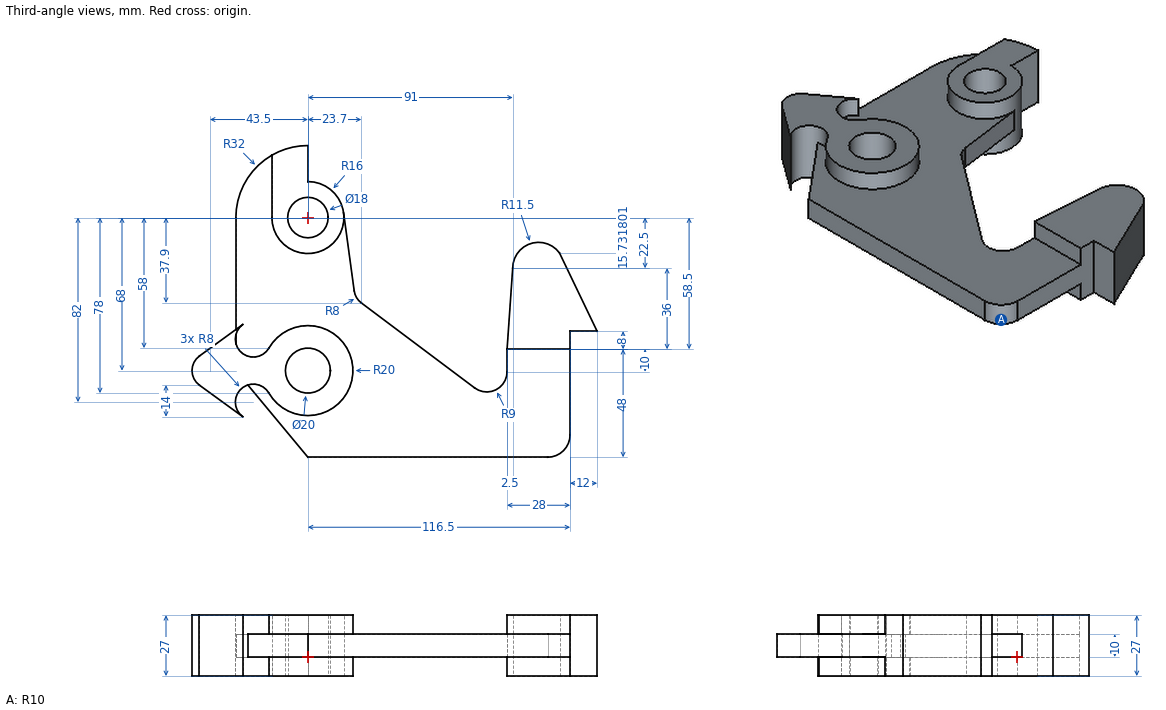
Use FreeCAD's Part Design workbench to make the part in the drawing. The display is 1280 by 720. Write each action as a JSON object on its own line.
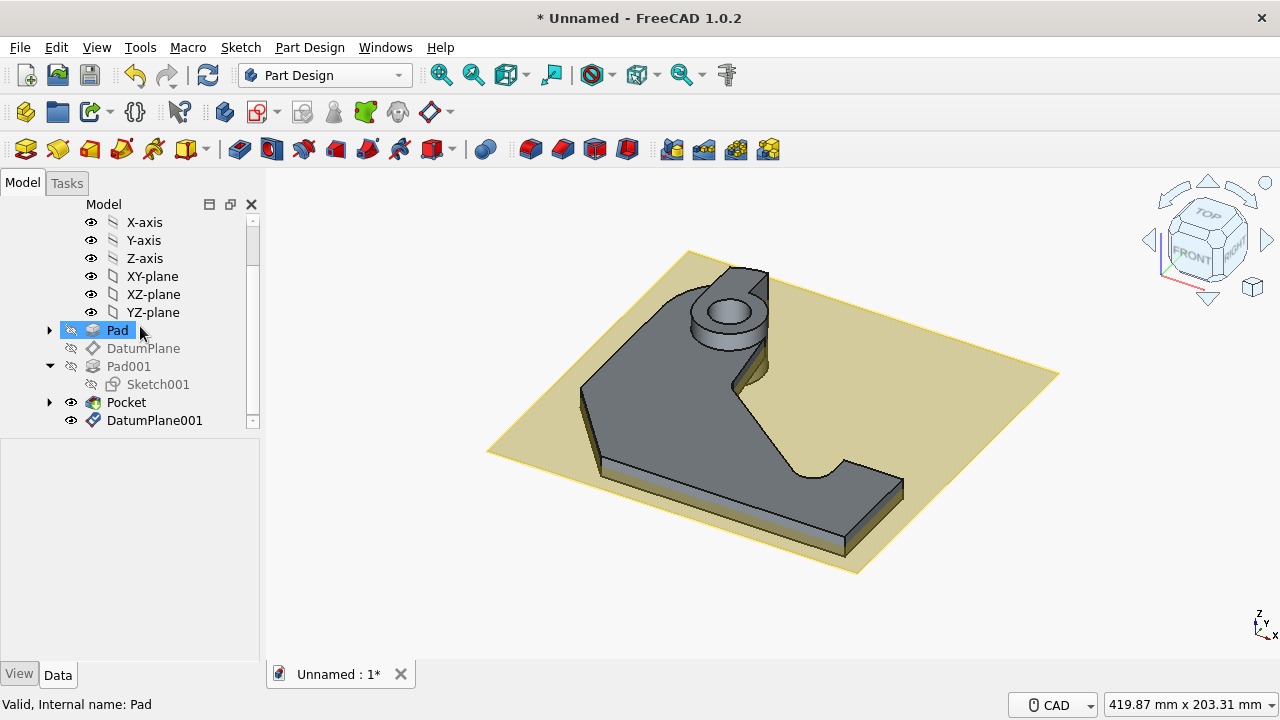
{"action": "left_click", "coordinate": [116, 420]}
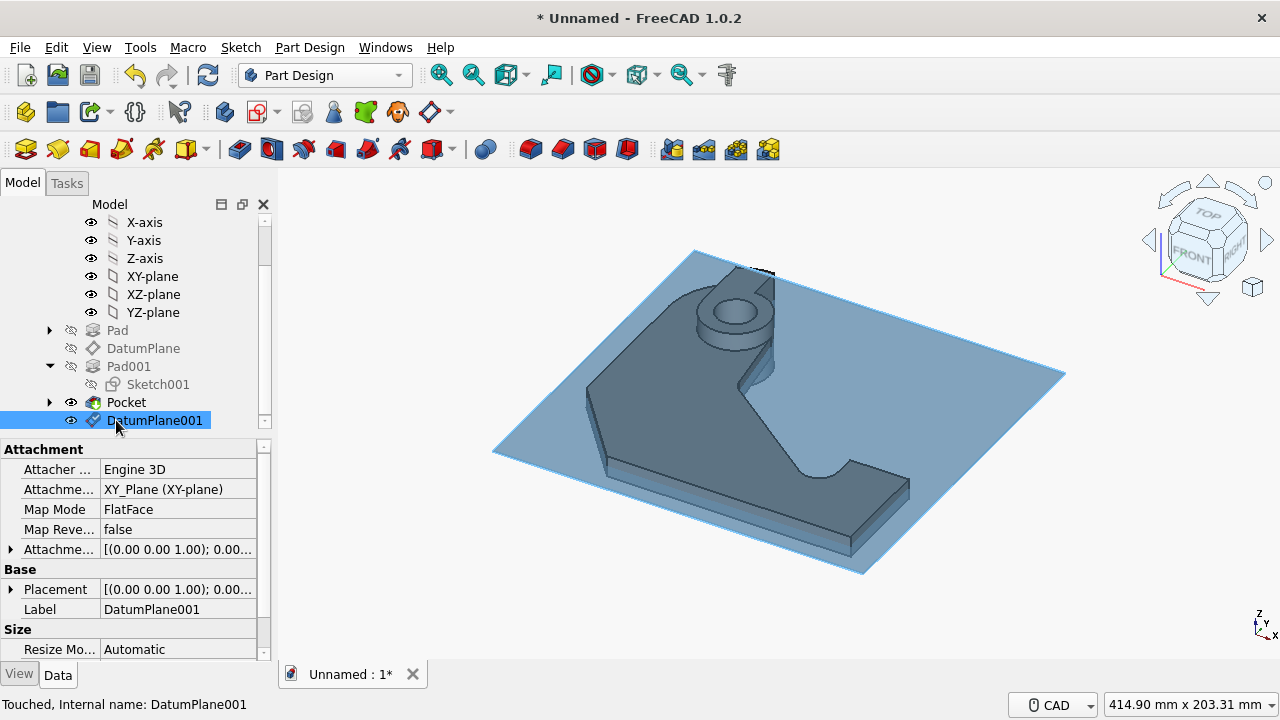
{"action": "left_click", "coordinate": [258, 112]}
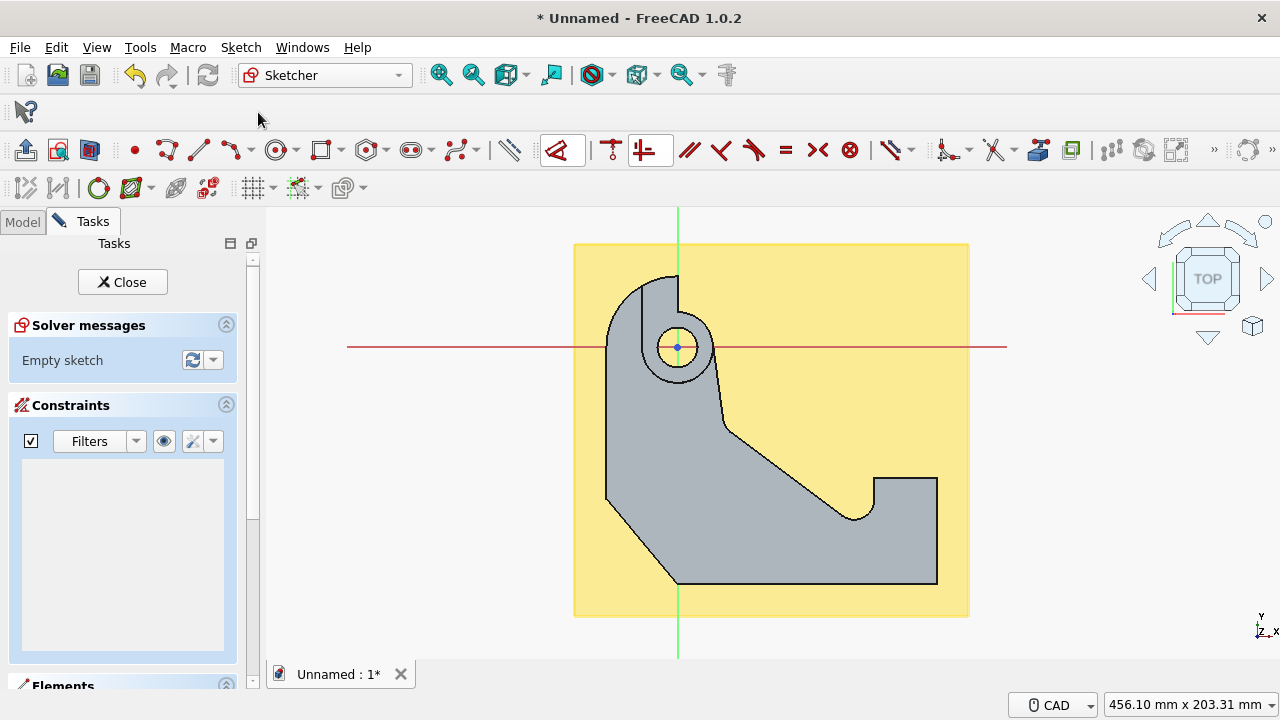
{"action": "left_click", "coordinate": [90, 150]}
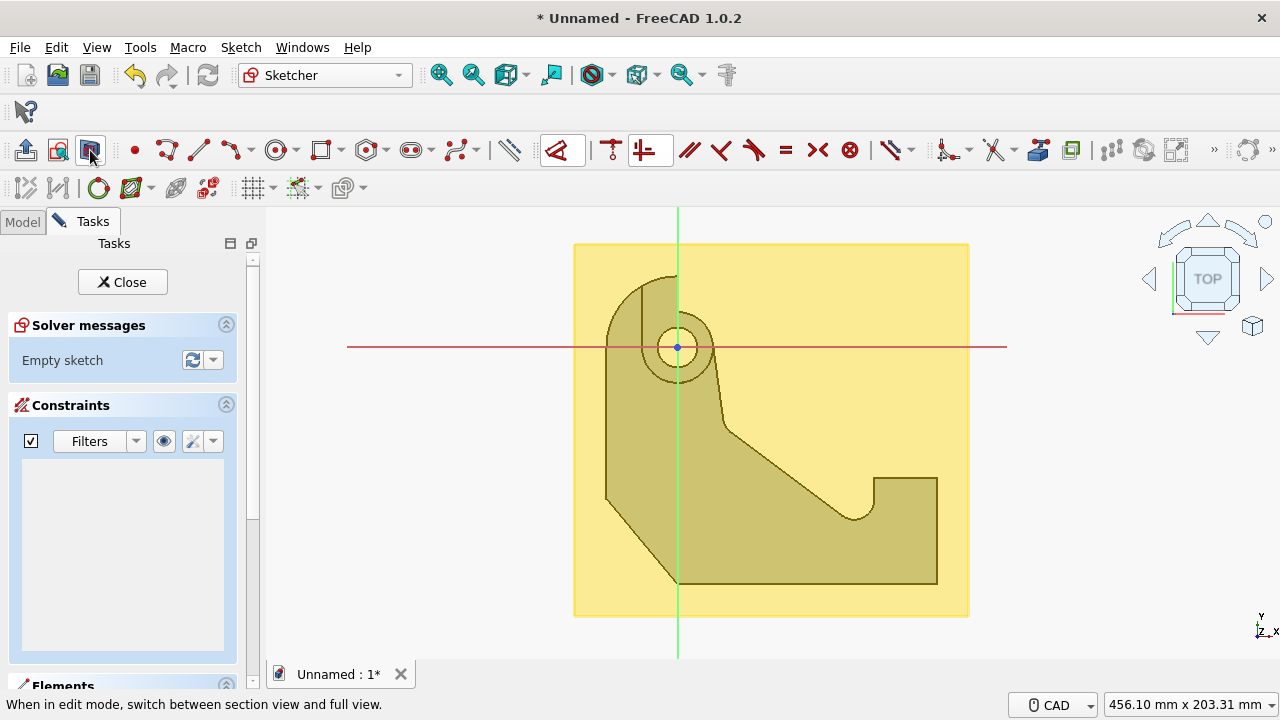
{"action": "scroll", "coordinate": [516, 472], "scroll_direction": "up", "scroll_amount": 2}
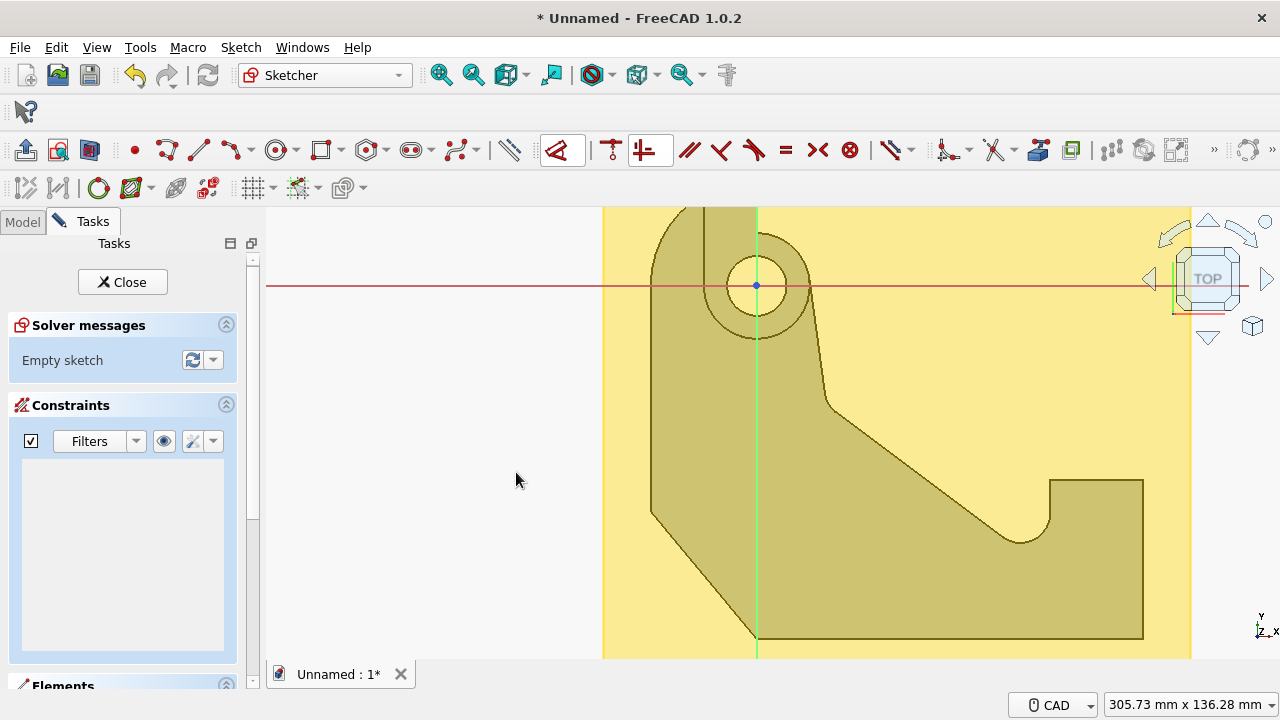
{"action": "left_click", "coordinate": [200, 150]}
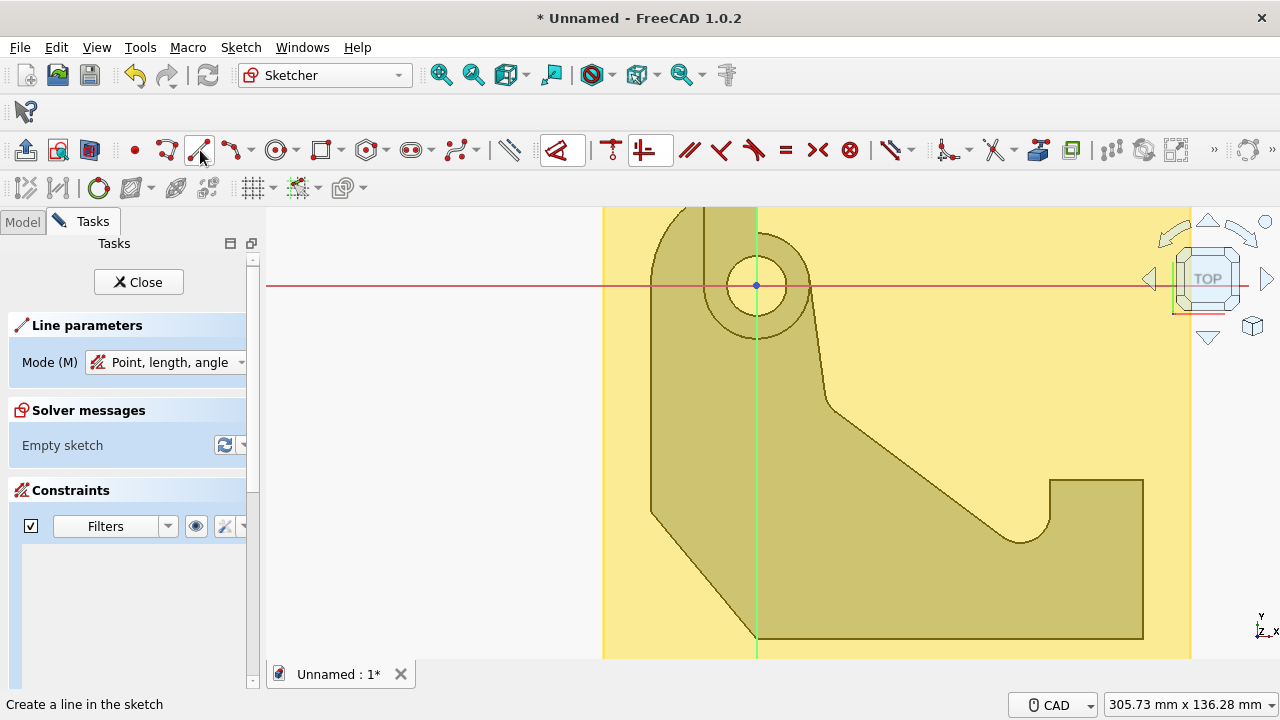
{"action": "left_click", "coordinate": [597, 533]}
{"action": "left_click", "coordinate": [661, 579]}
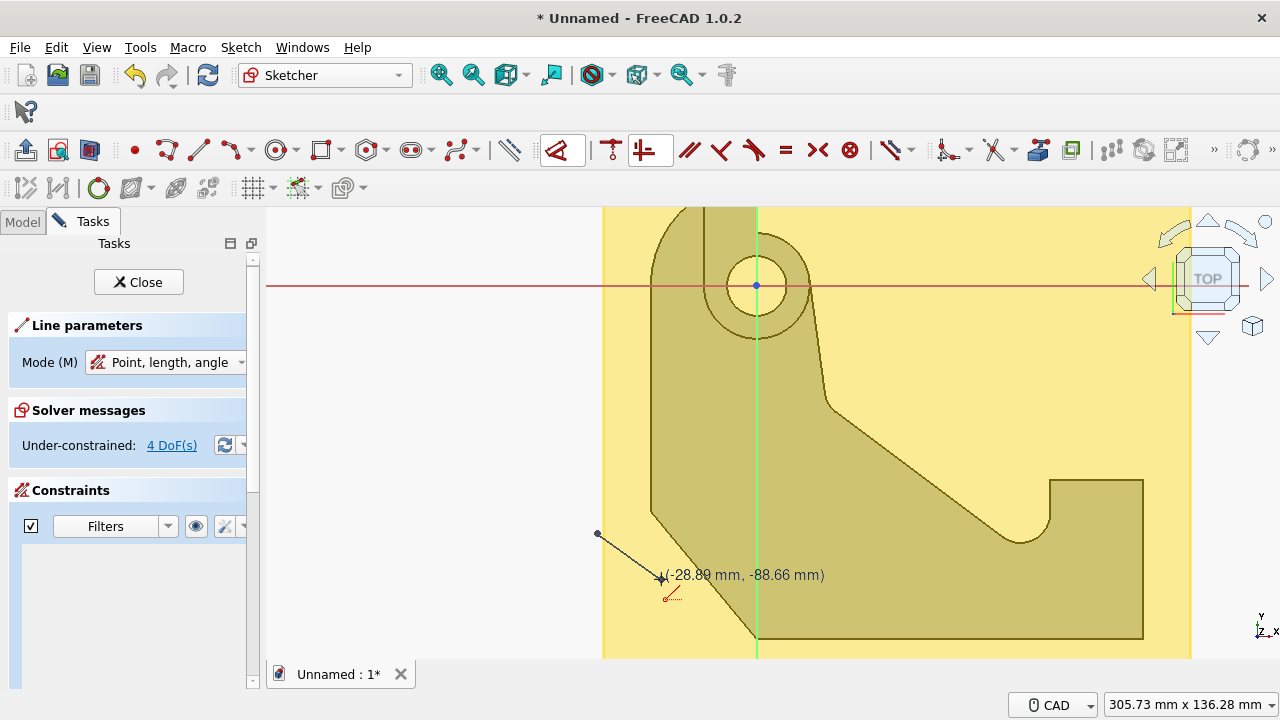
{"action": "left_click", "coordinate": [661, 444]}
{"action": "left_click", "coordinate": [597, 490]}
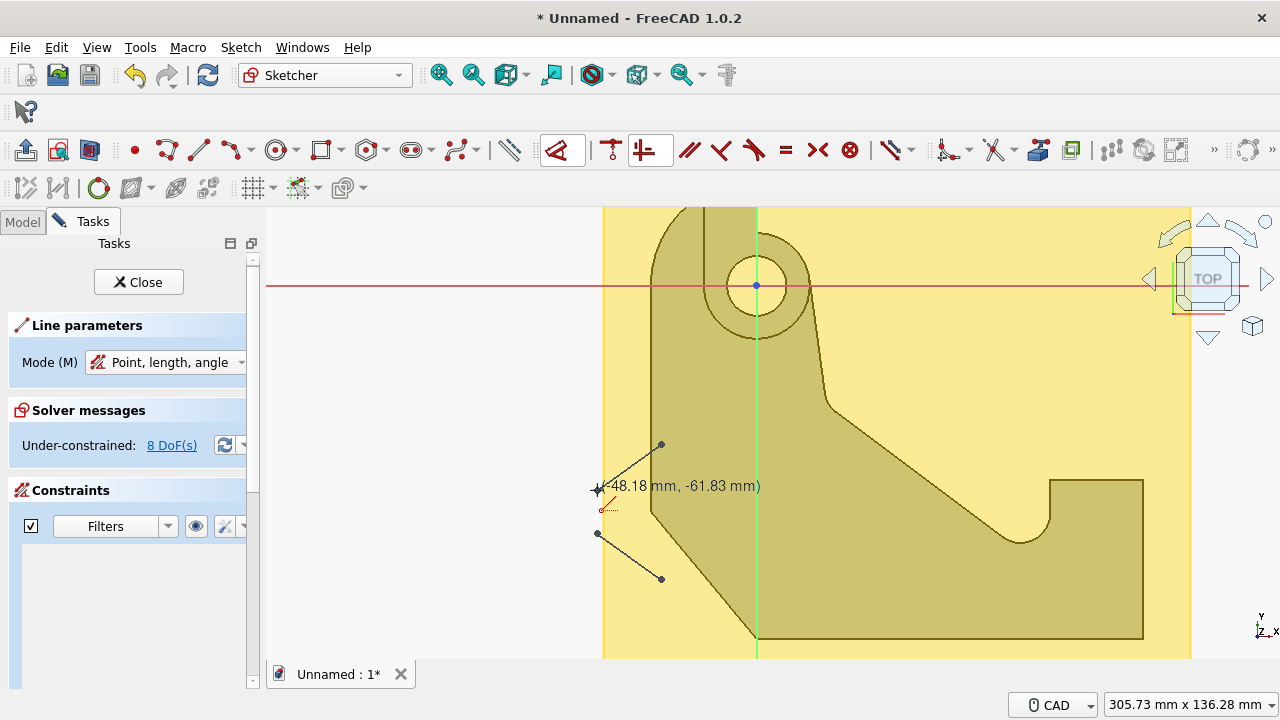
{"action": "key", "text": "g 3 a"}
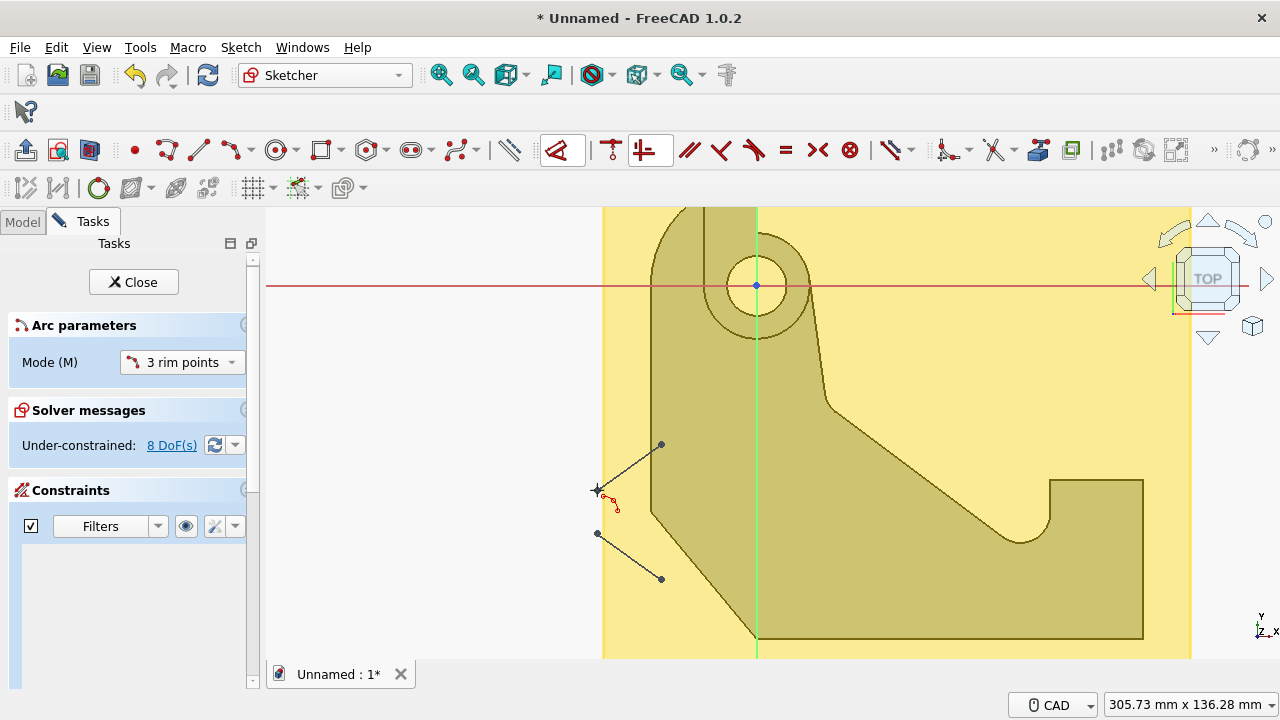
{"action": "left_click", "coordinate": [661, 580]}
{"action": "left_click", "coordinate": [699, 545]}
{"action": "left_click", "coordinate": [659, 538]}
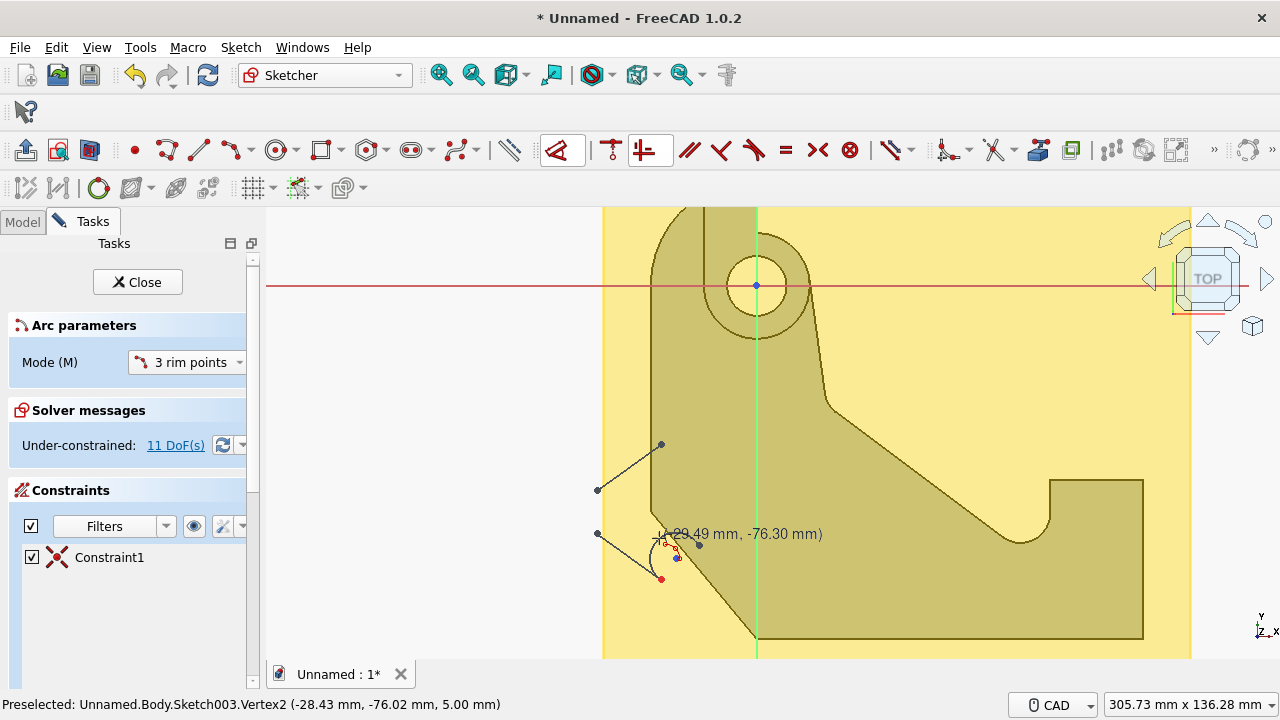
{"action": "left_click", "coordinate": [699, 546]}
{"action": "left_click", "coordinate": [699, 478]}
{"action": "left_click", "coordinate": [823, 511]}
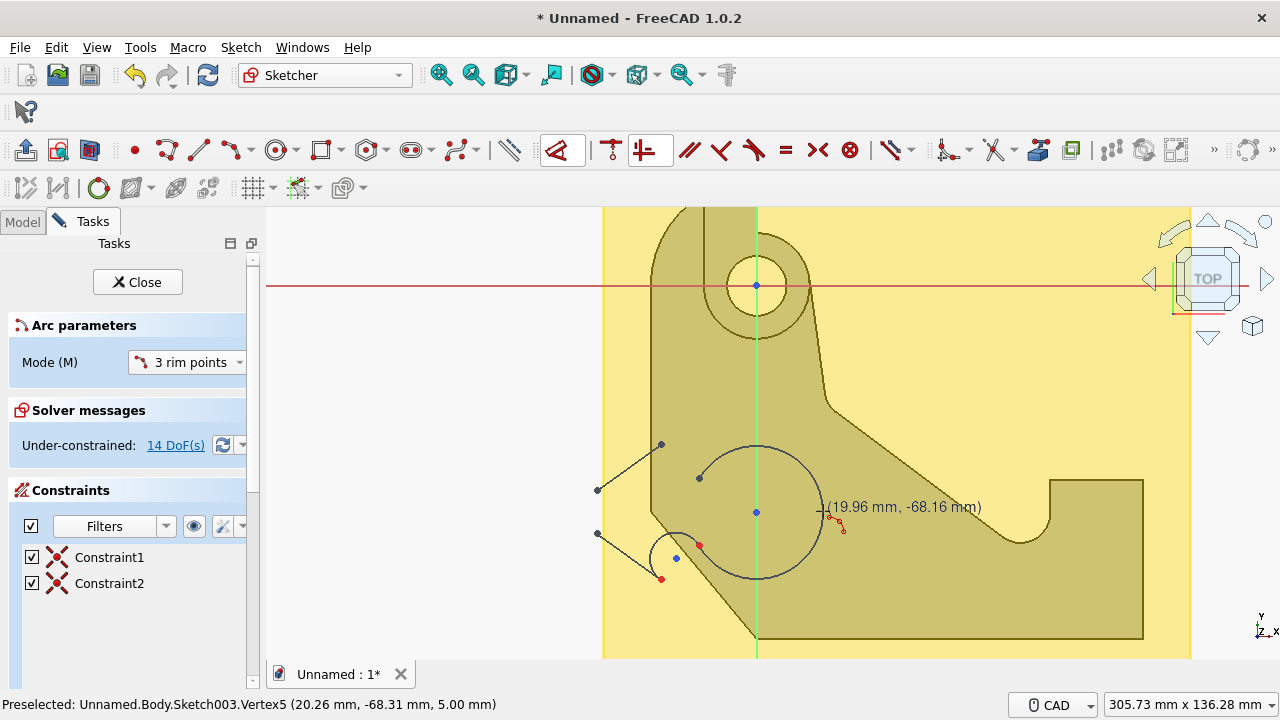
{"action": "left_click", "coordinate": [699, 479]}
{"action": "left_click", "coordinate": [661, 445]}
{"action": "left_click", "coordinate": [659, 485]}